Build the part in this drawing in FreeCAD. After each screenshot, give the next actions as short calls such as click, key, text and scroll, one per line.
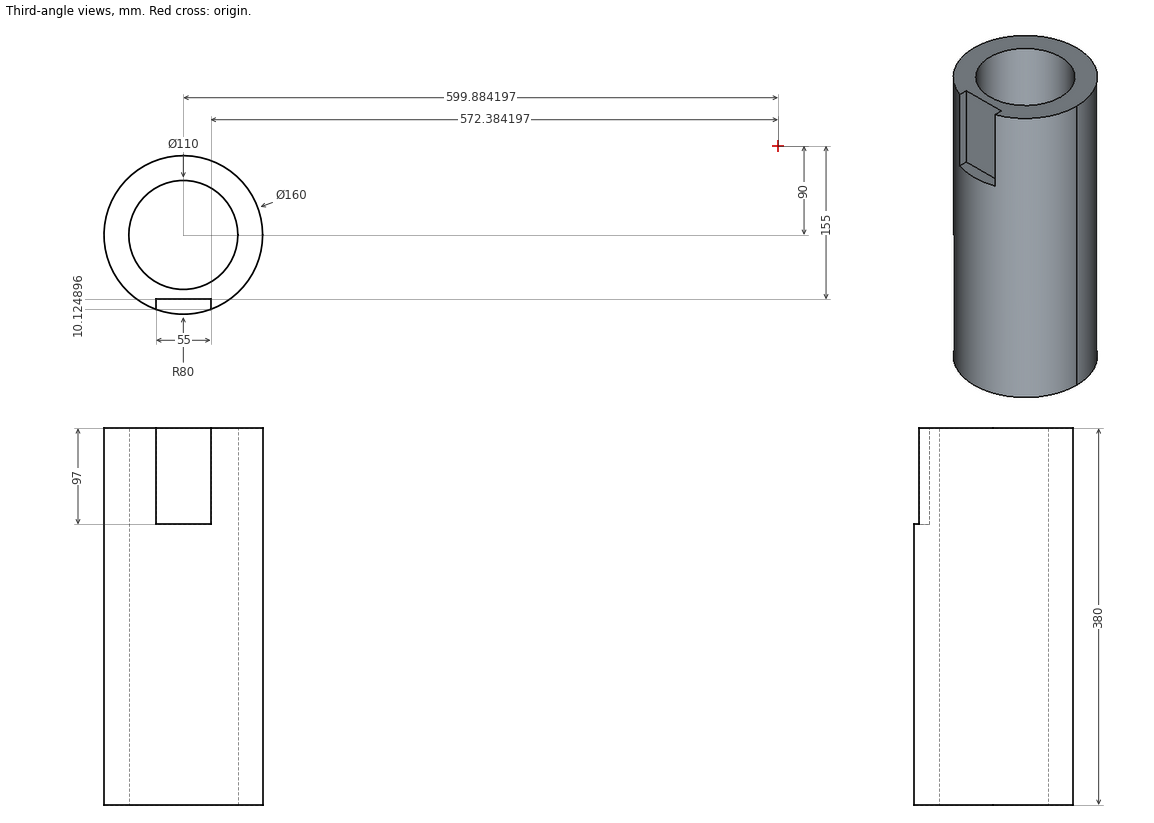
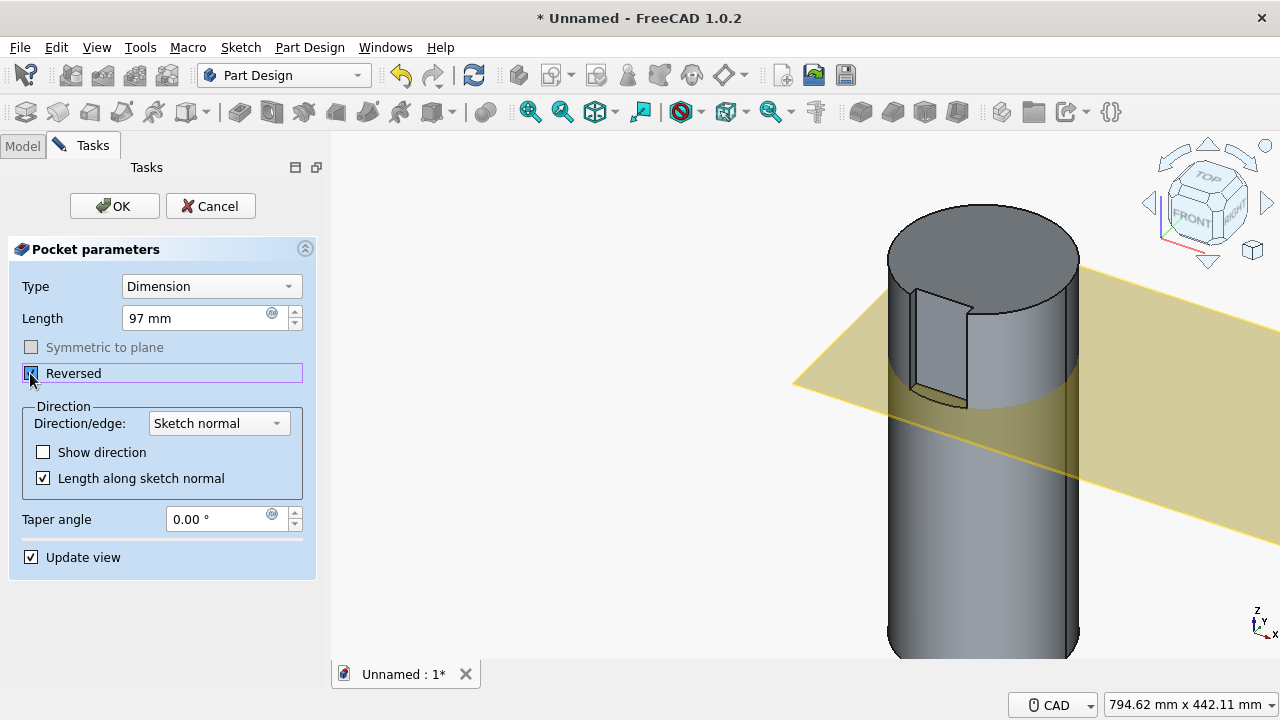
click(115, 206)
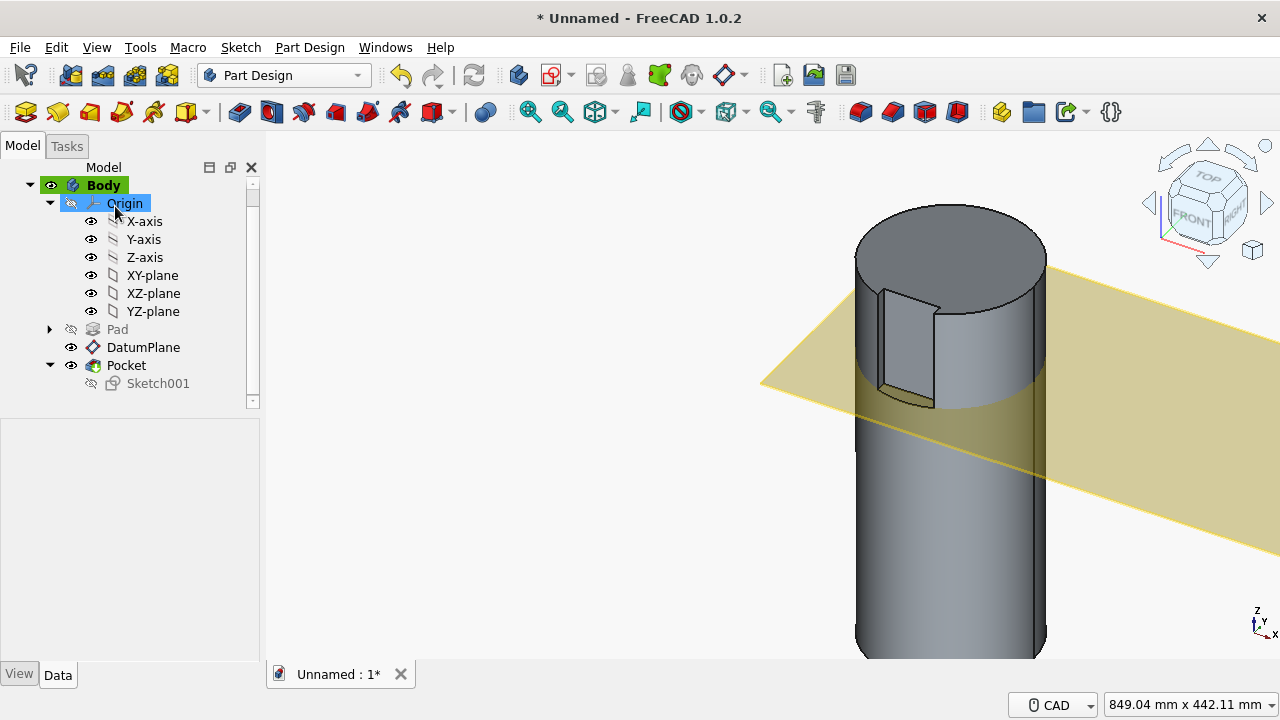
click(116, 347)
key(space)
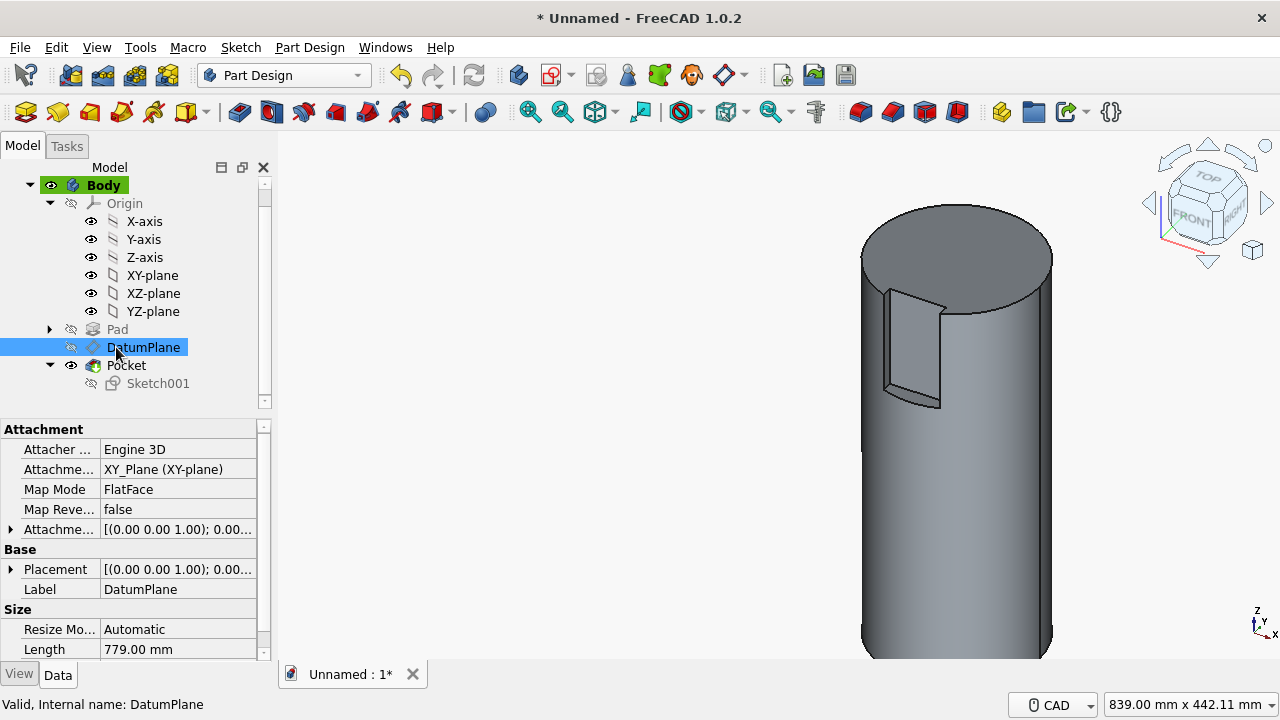
click(532, 112)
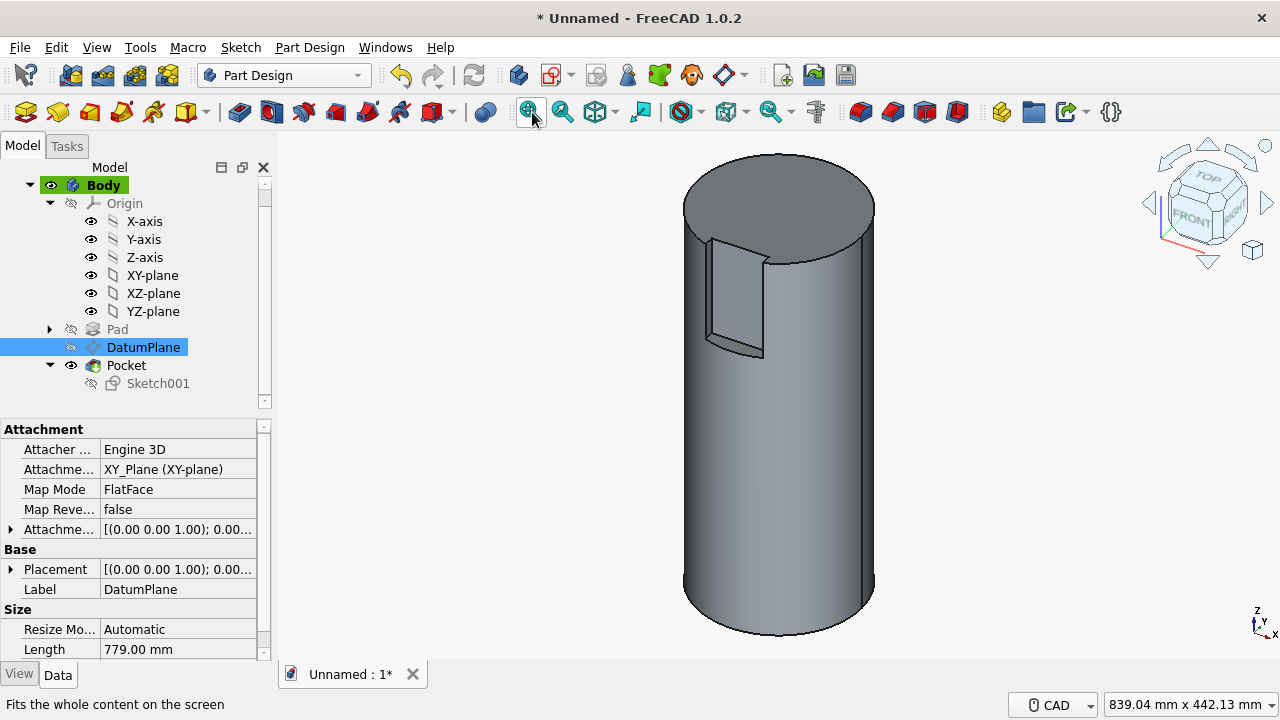
click(780, 207)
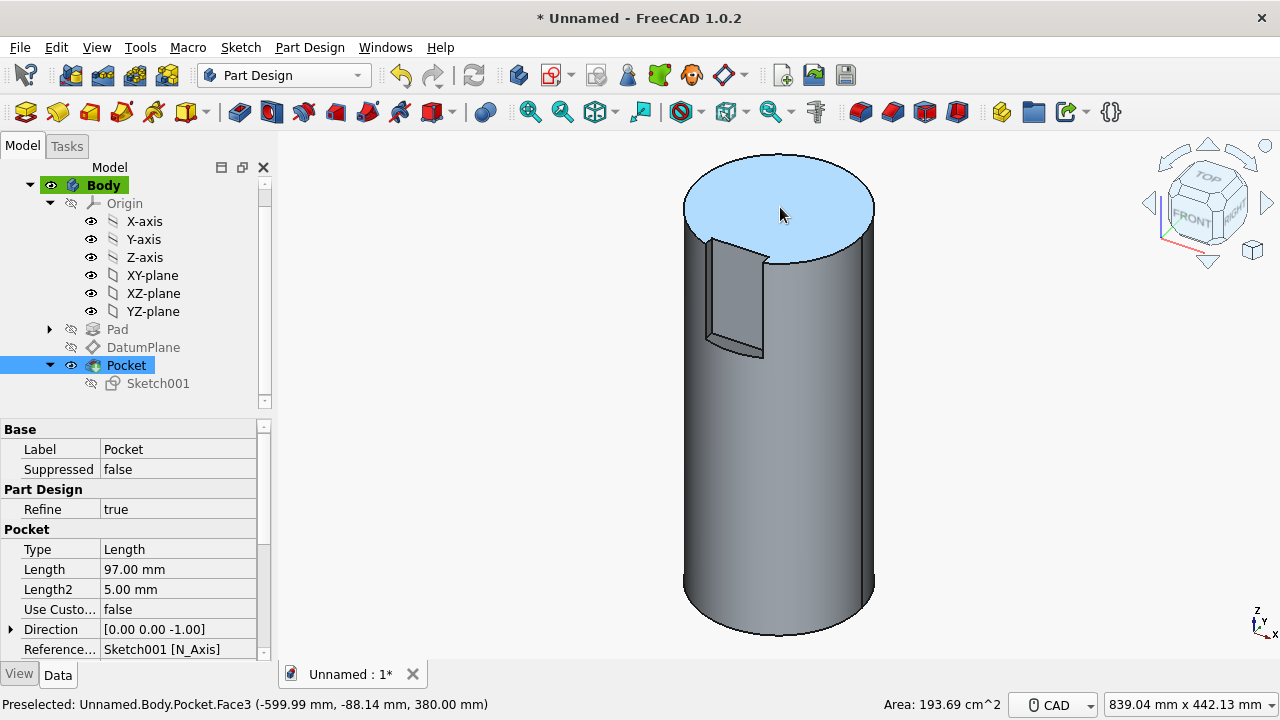
click(552, 76)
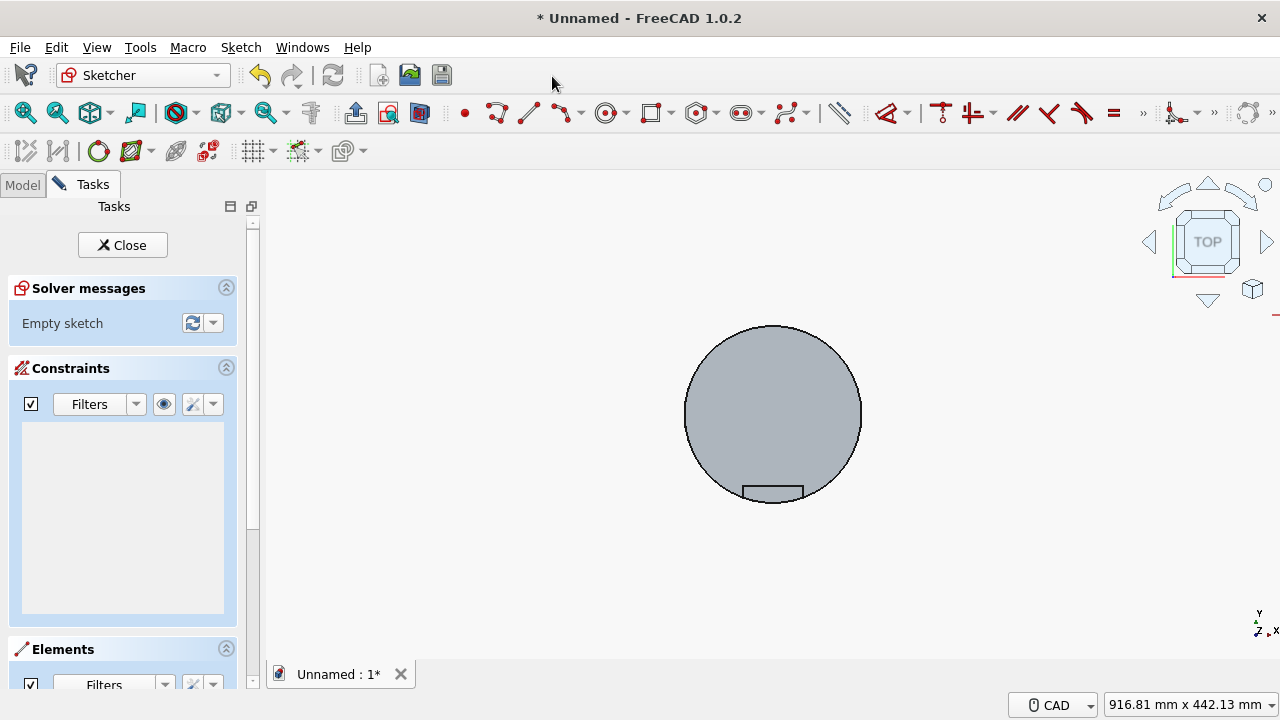
scroll(813, 415, up, 5)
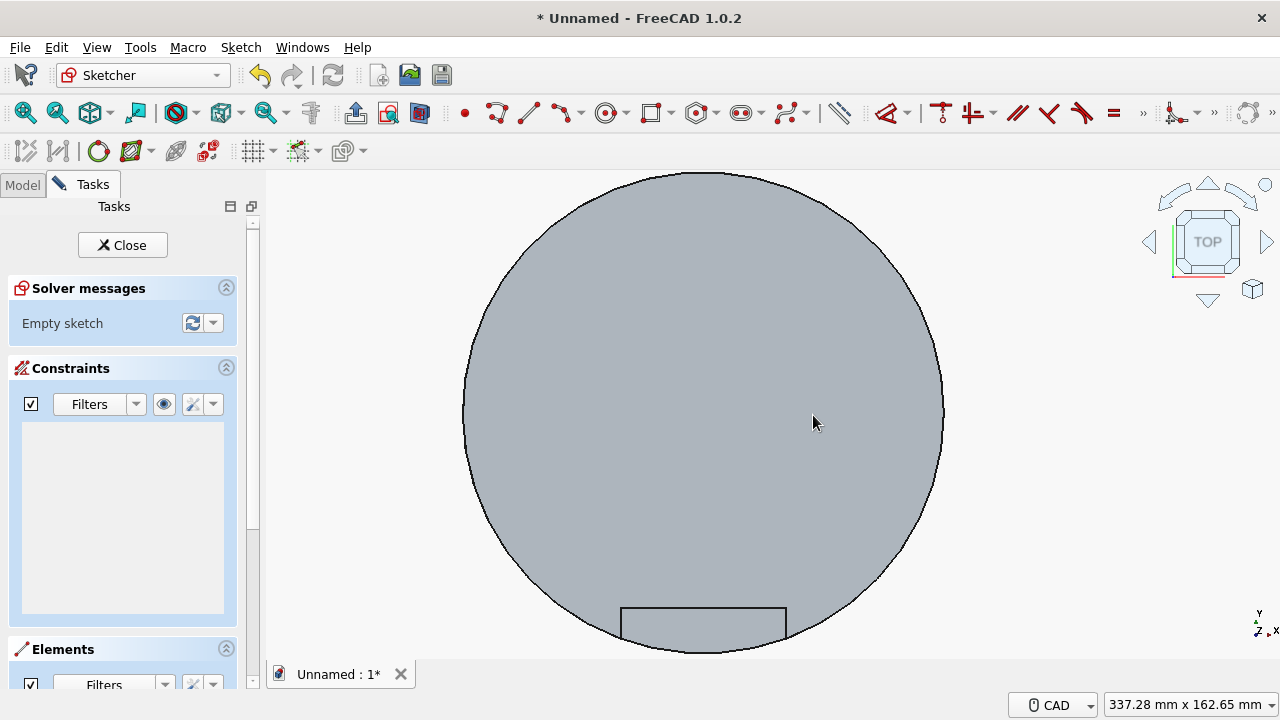
click(606, 114)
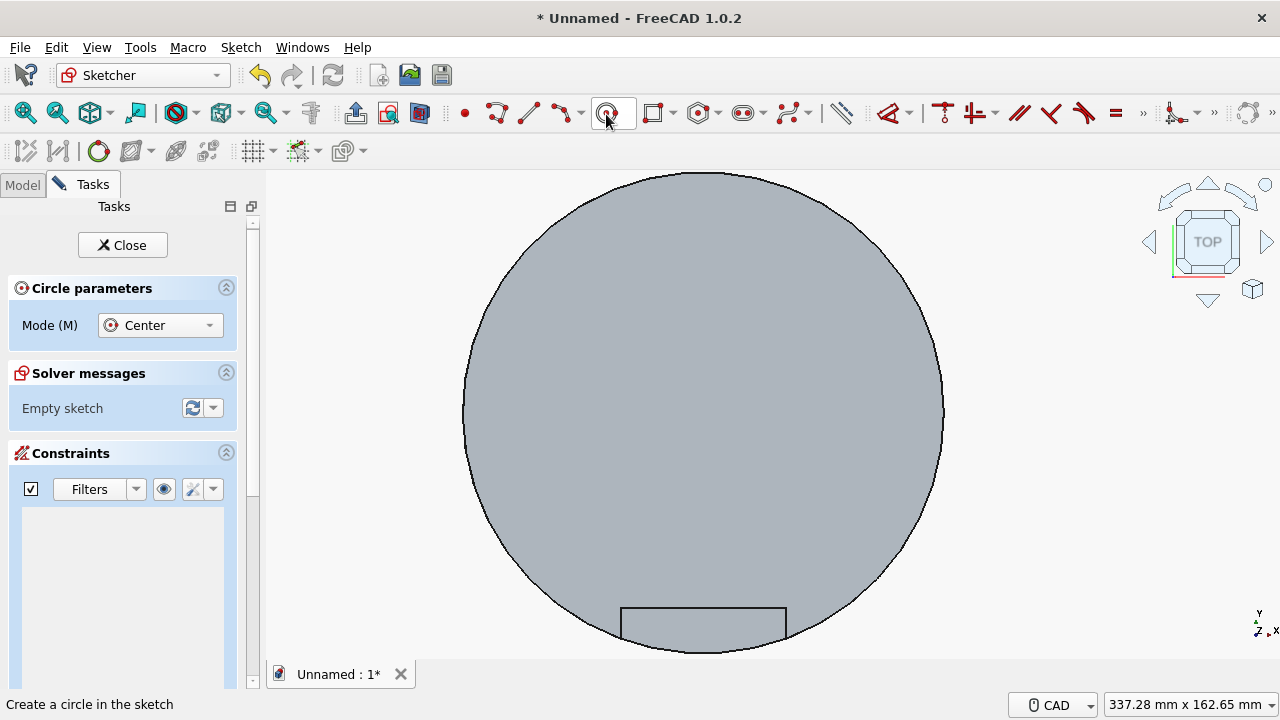
click(703, 413)
click(820, 296)
key(Escape)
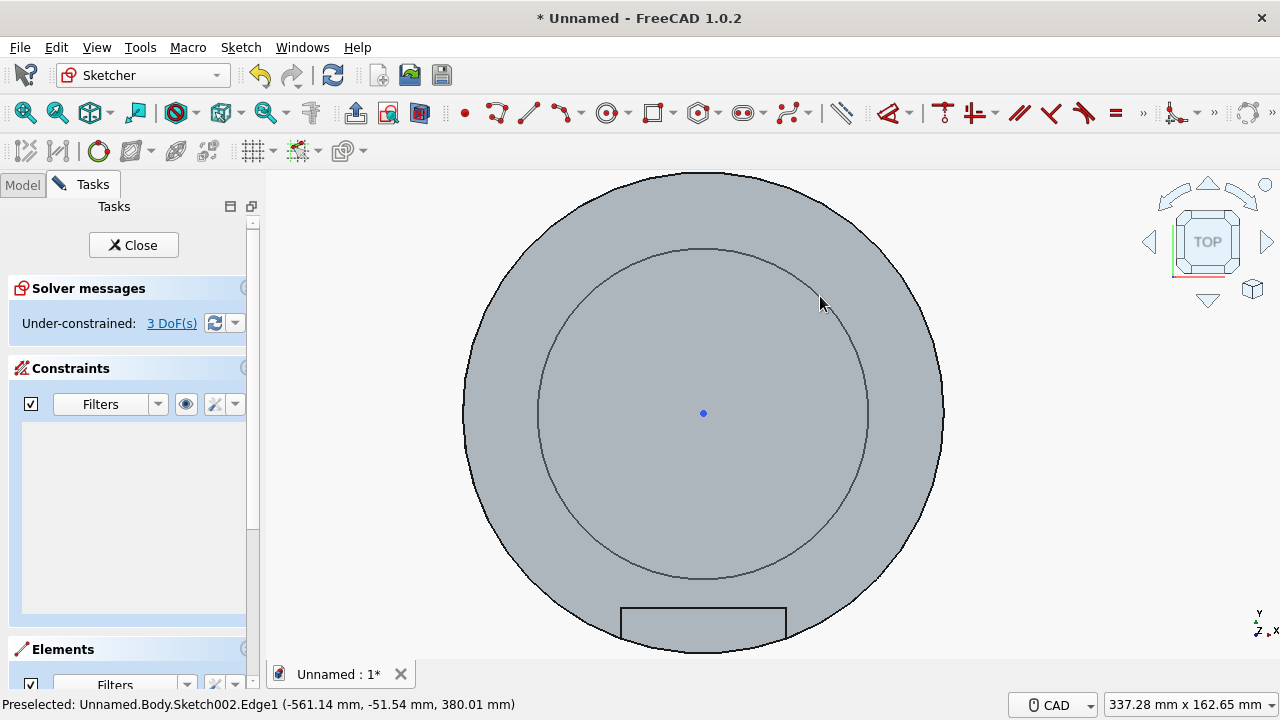
click(888, 114)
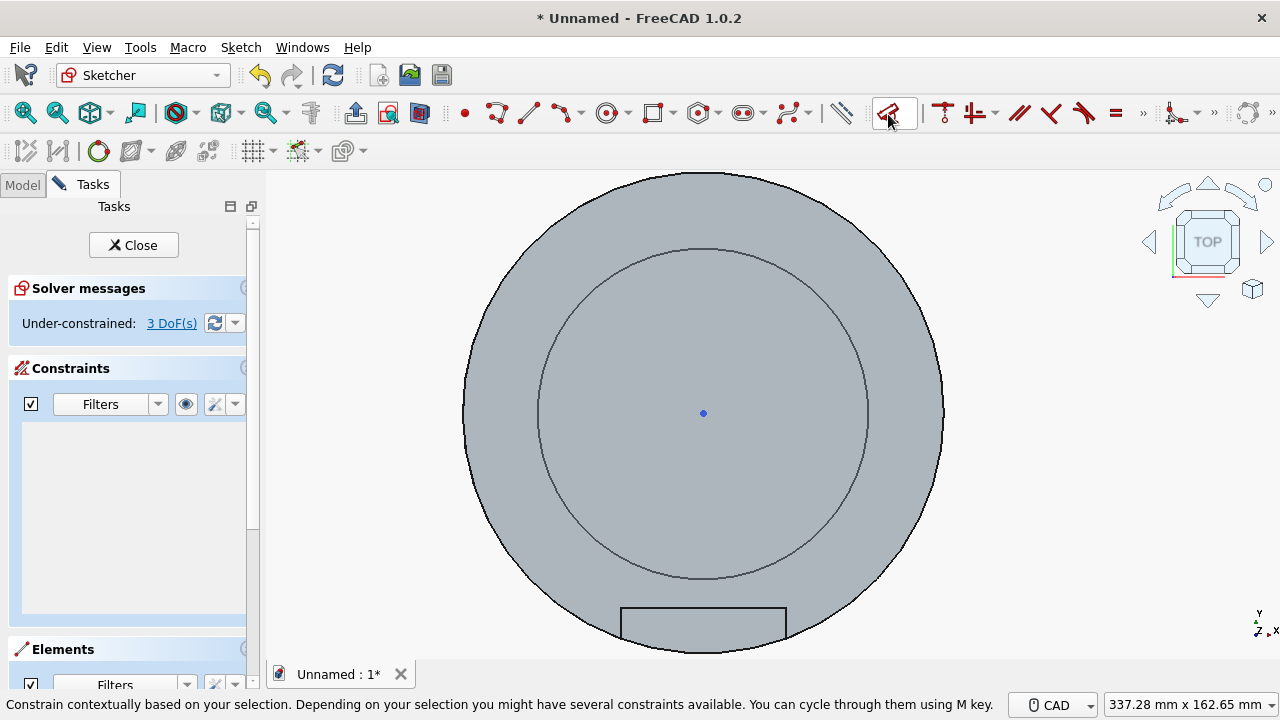
click(820, 297)
click(843, 274)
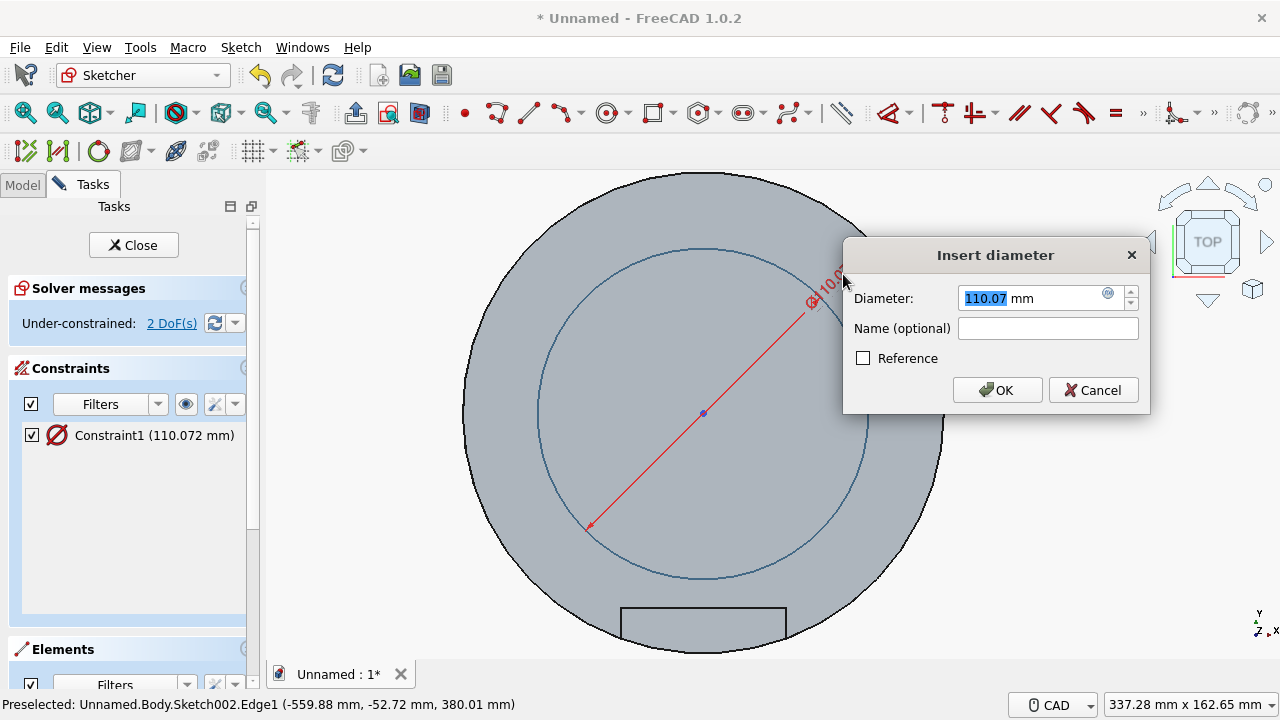
text(110)
key(Return)